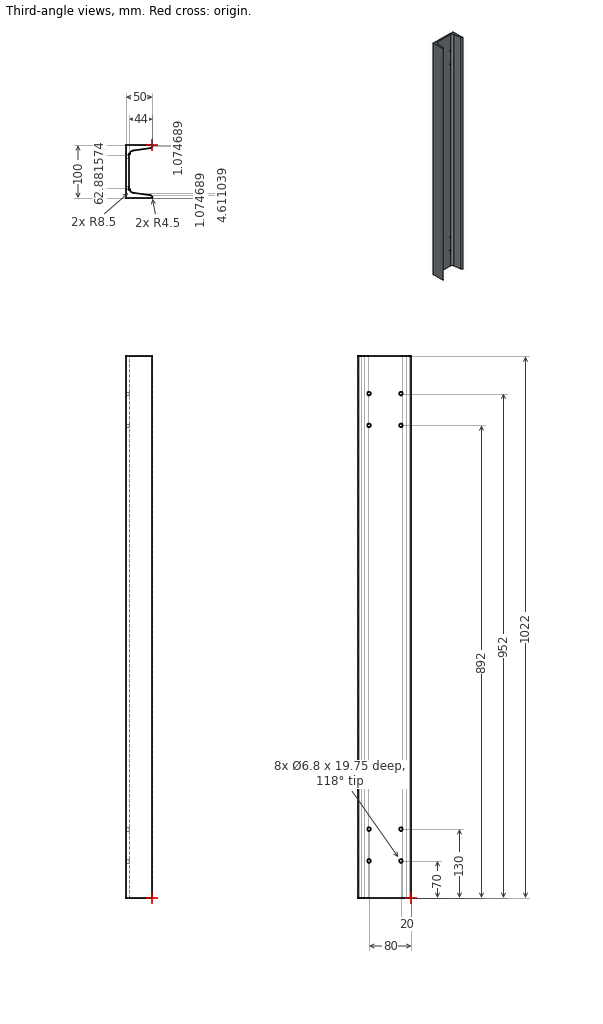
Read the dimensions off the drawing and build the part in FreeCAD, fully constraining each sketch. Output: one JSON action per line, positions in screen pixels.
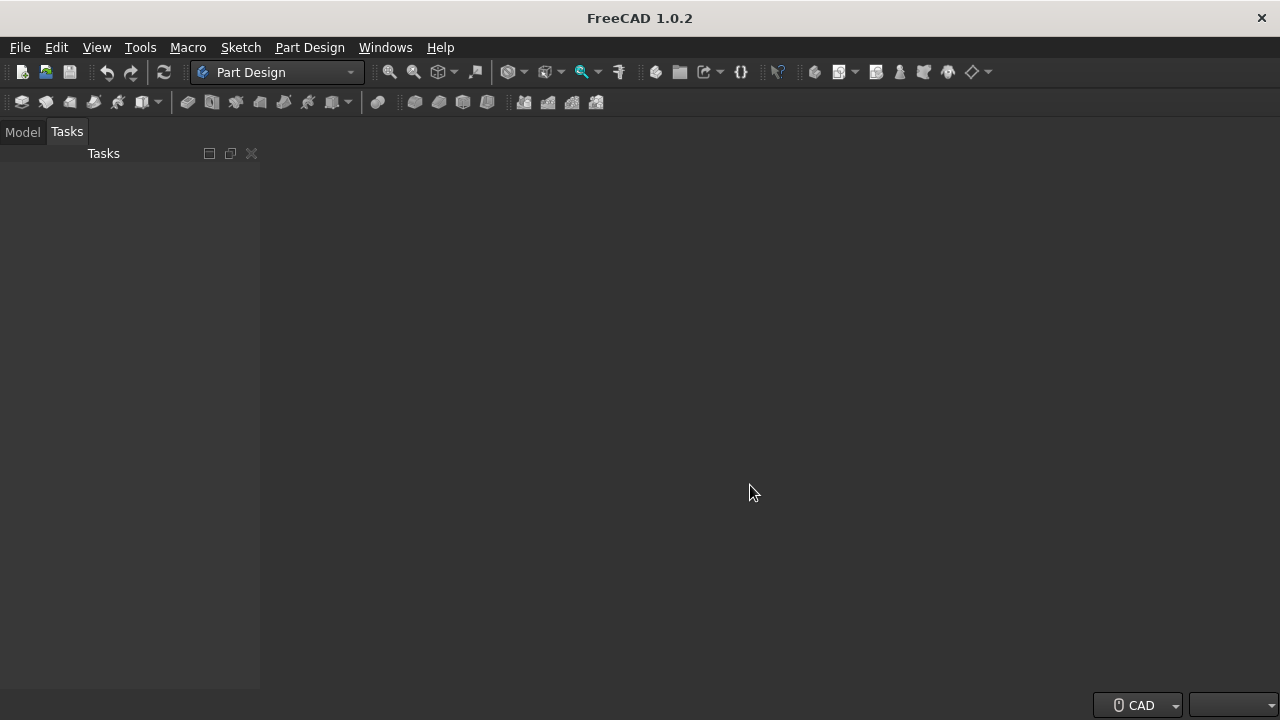
{"action": "left_click", "coordinate": [22, 72]}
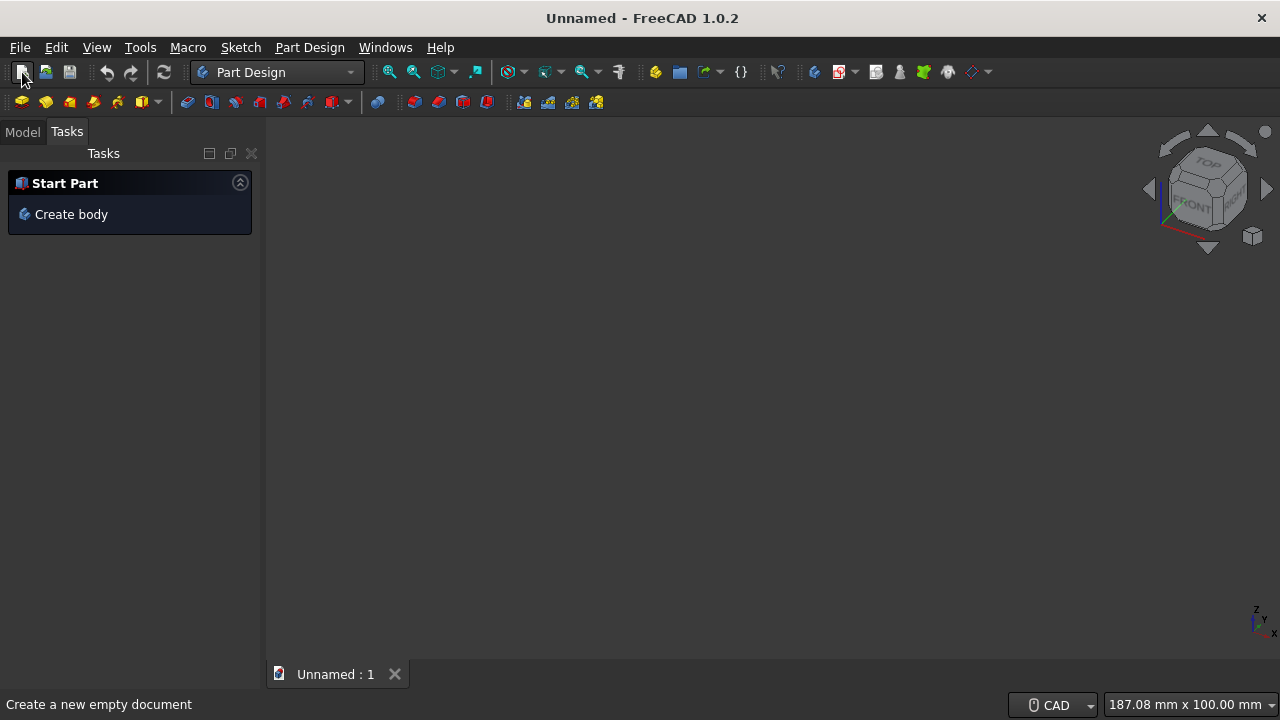
{"action": "left_click", "coordinate": [840, 72]}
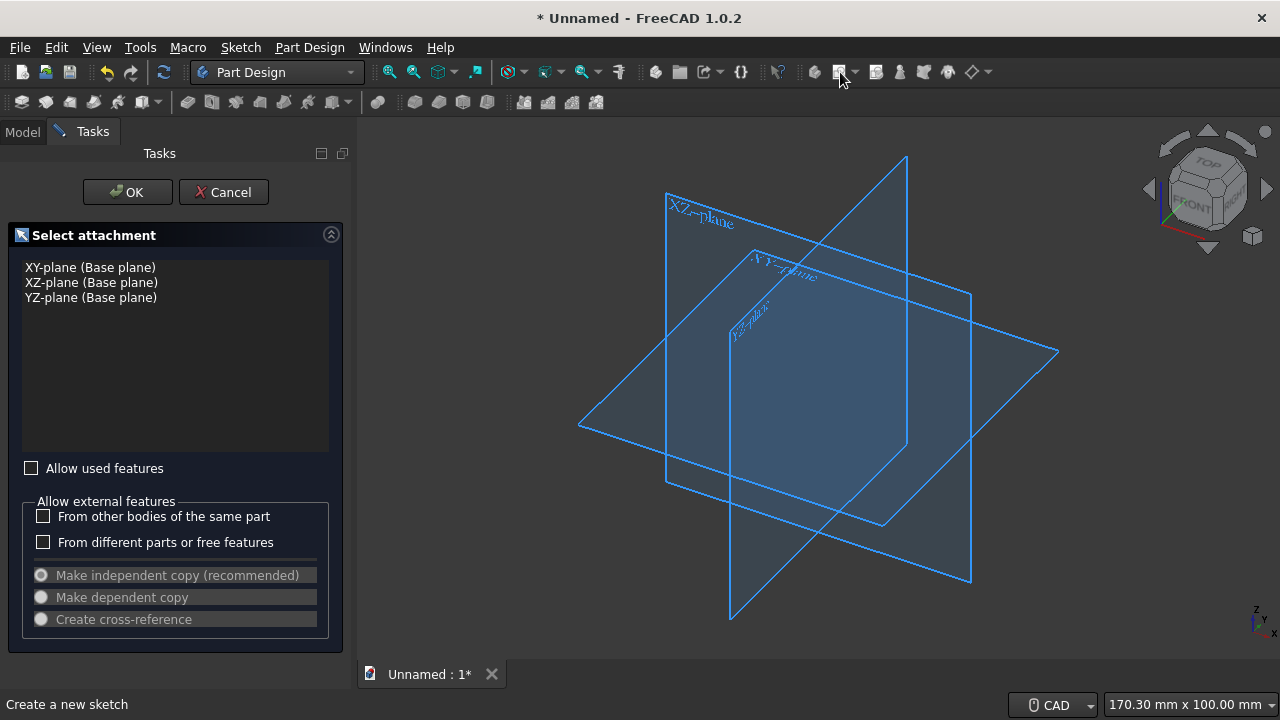
{"action": "left_click", "coordinate": [82, 268]}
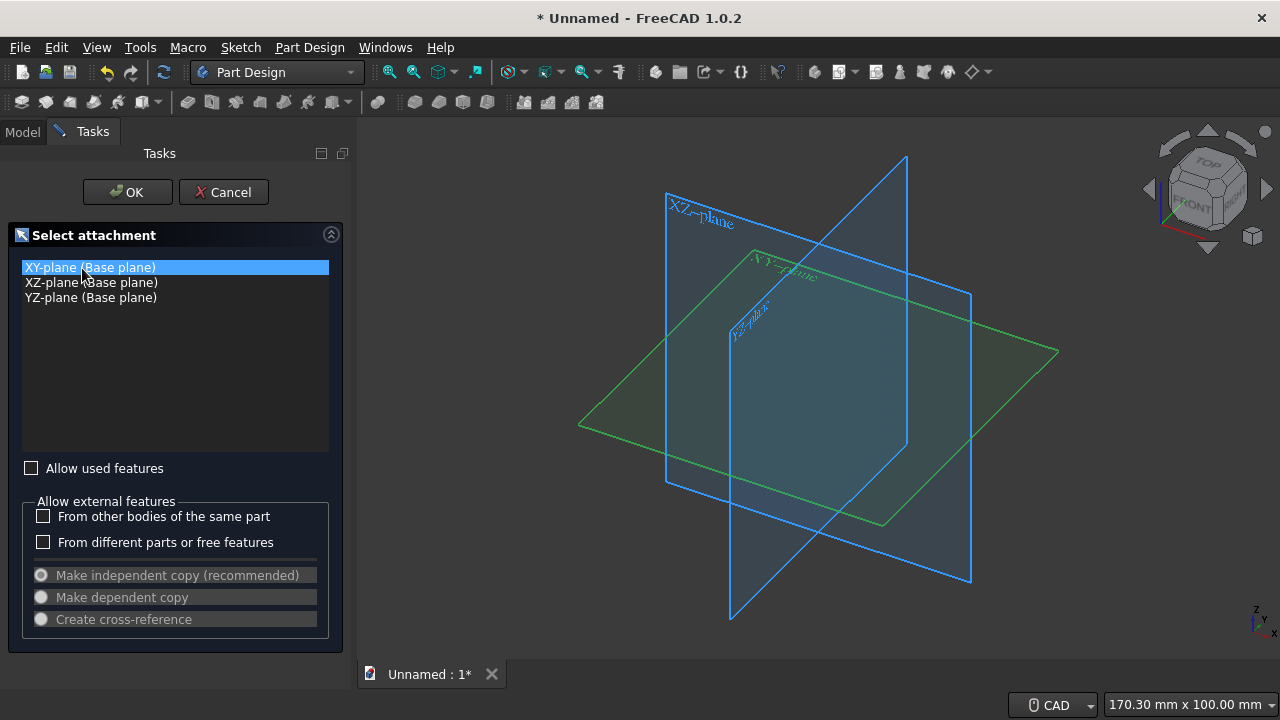
{"action": "left_click", "coordinate": [128, 192]}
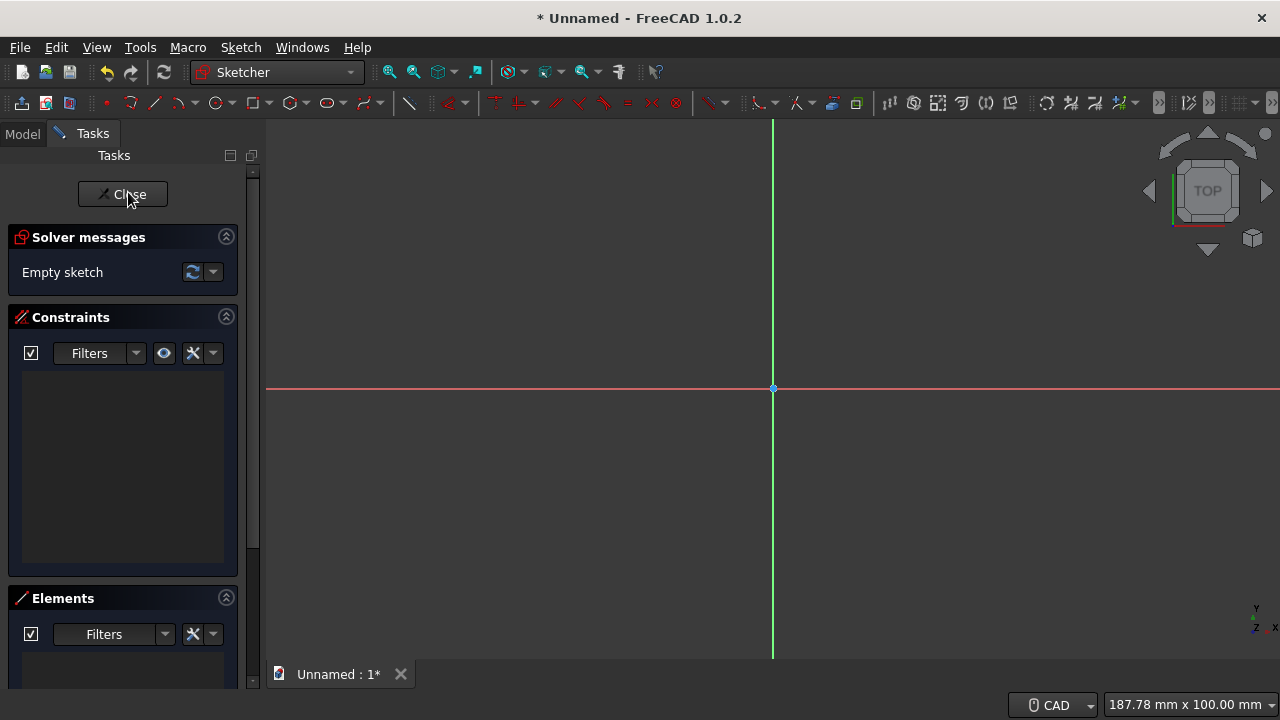
{"action": "scroll", "coordinate": [785, 147], "scroll_direction": "down", "scroll_amount": 3}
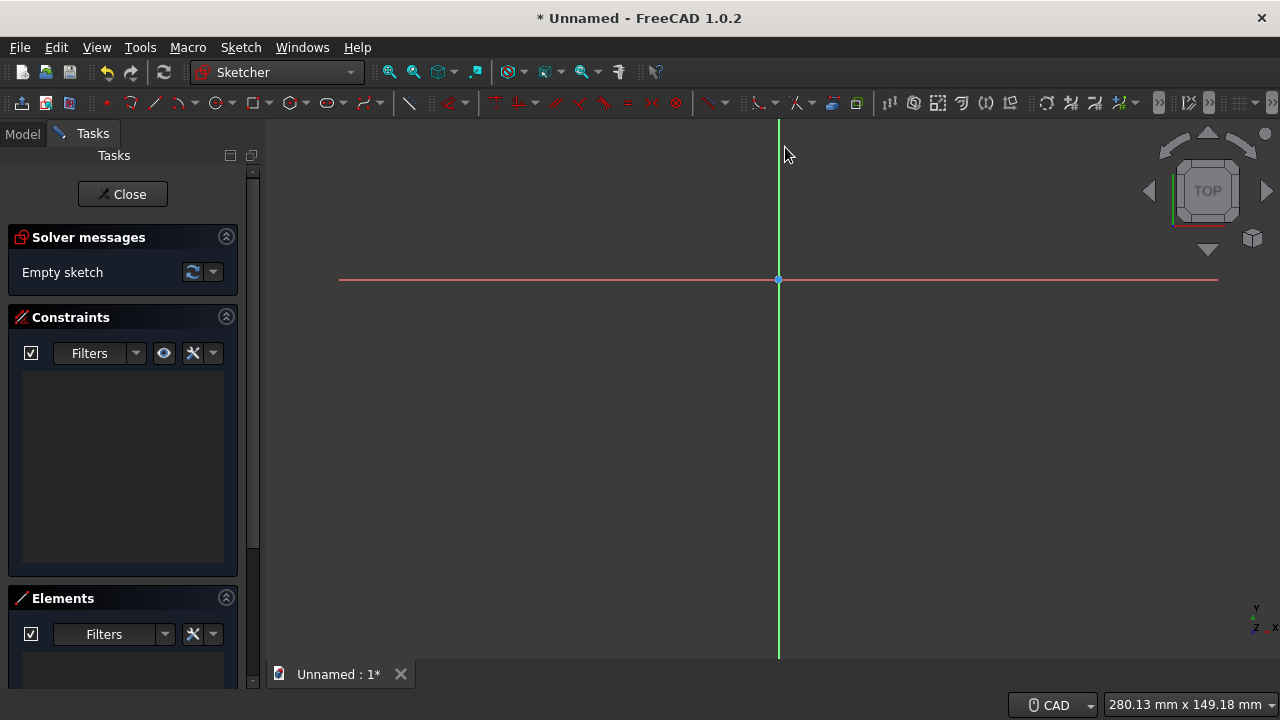
{"action": "left_click", "coordinate": [156, 104]}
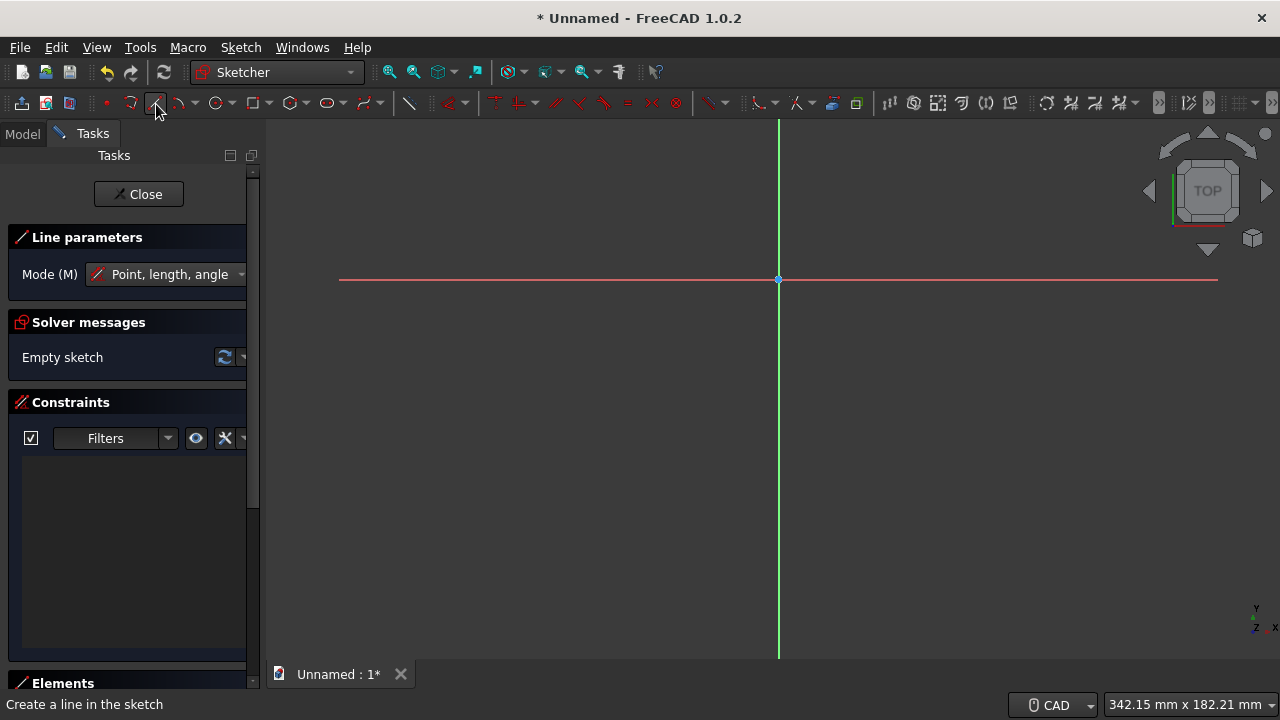
{"action": "scroll", "coordinate": [767, 560], "scroll_direction": "up", "scroll_amount": 2}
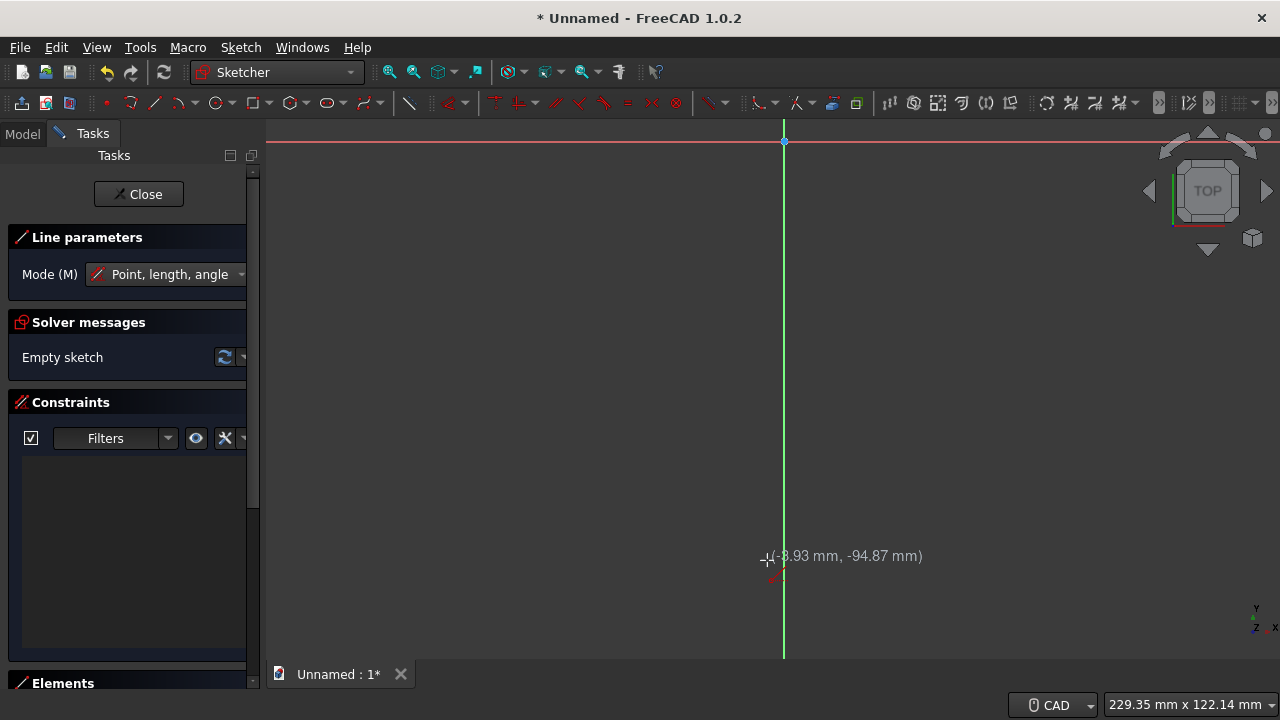
{"action": "left_click", "coordinate": [767, 559]}
{"action": "left_click", "coordinate": [622, 539]}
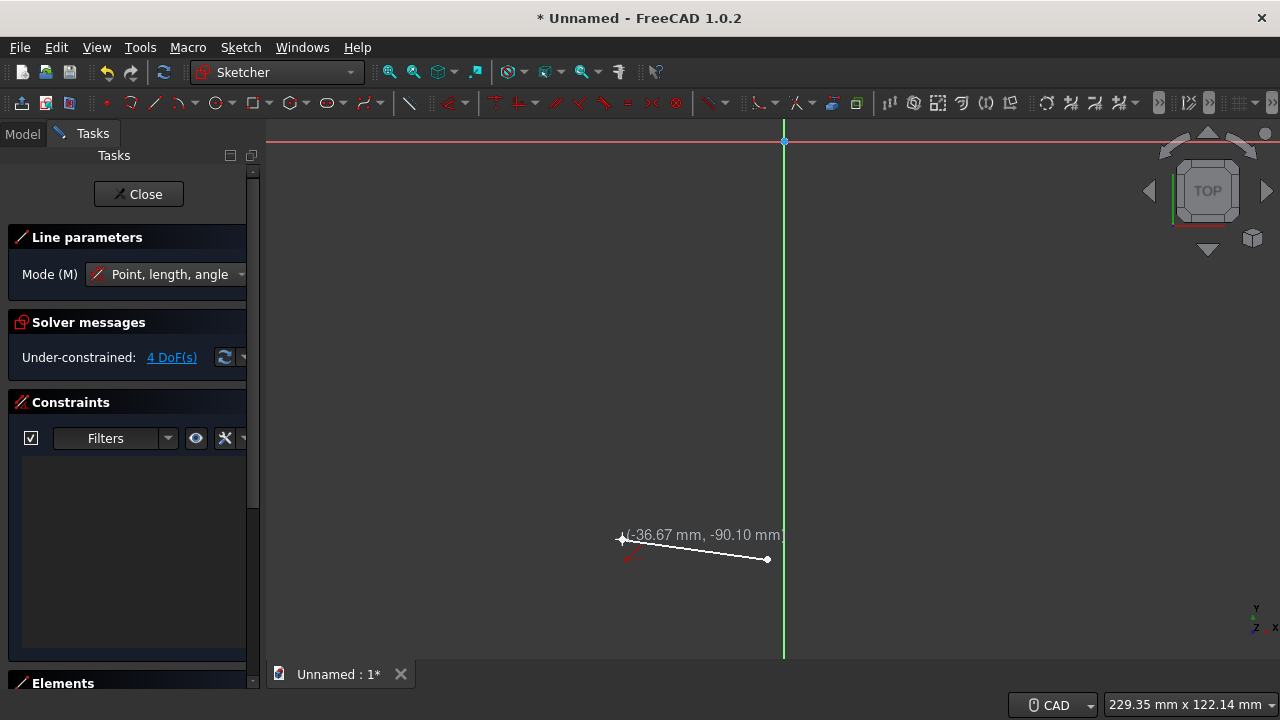
{"action": "left_click", "coordinate": [590, 502]}
{"action": "left_click", "coordinate": [590, 224]}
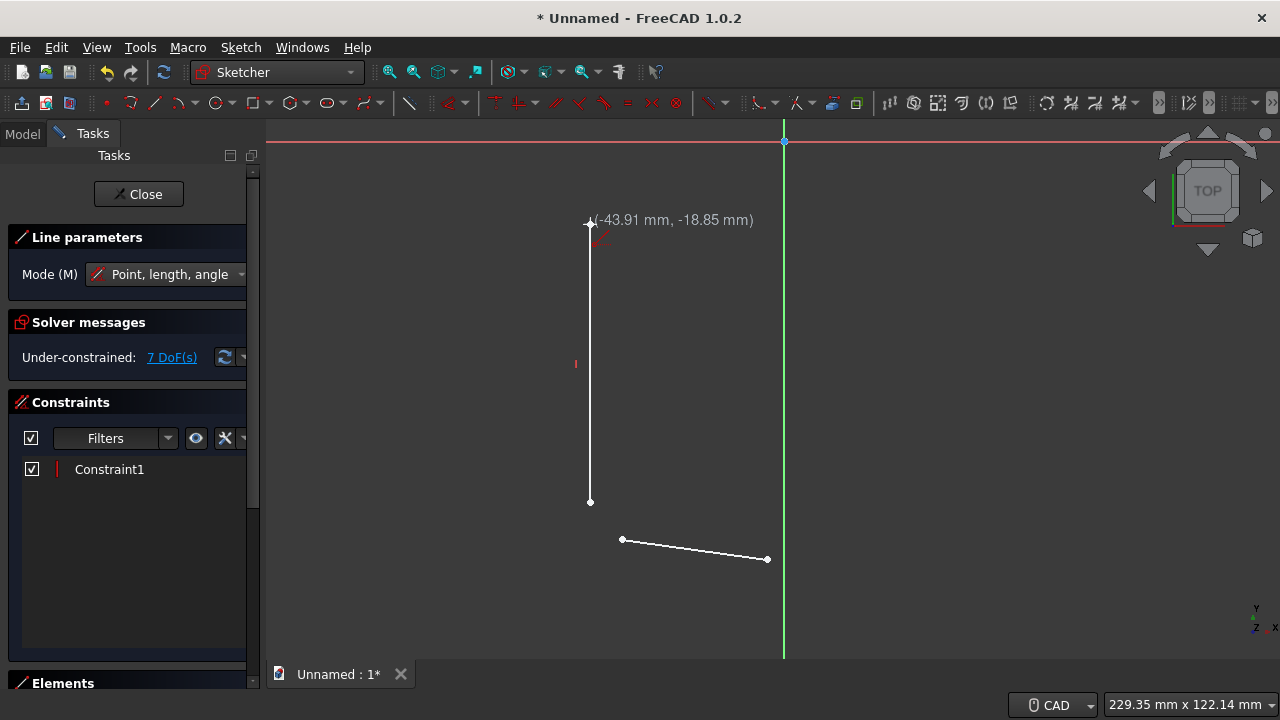
{"action": "left_click", "coordinate": [622, 186]}
{"action": "left_click", "coordinate": [767, 166]}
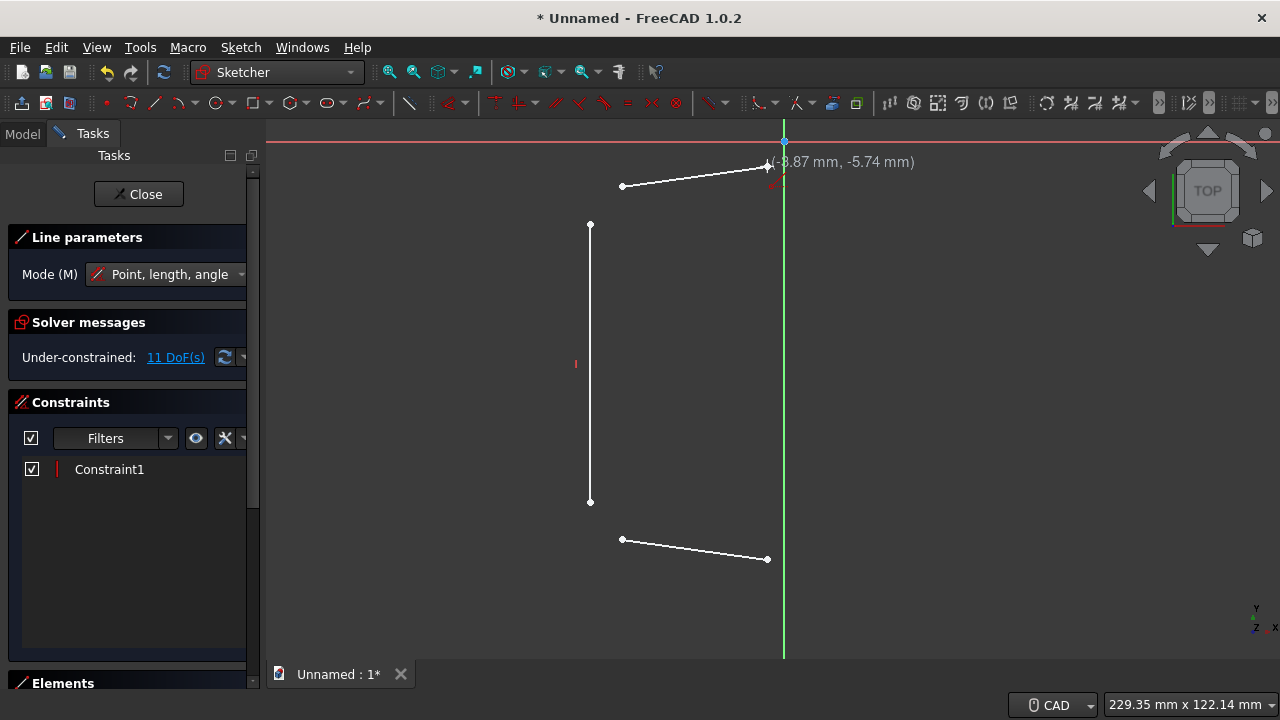
{"action": "left_click", "coordinate": [132, 104]}